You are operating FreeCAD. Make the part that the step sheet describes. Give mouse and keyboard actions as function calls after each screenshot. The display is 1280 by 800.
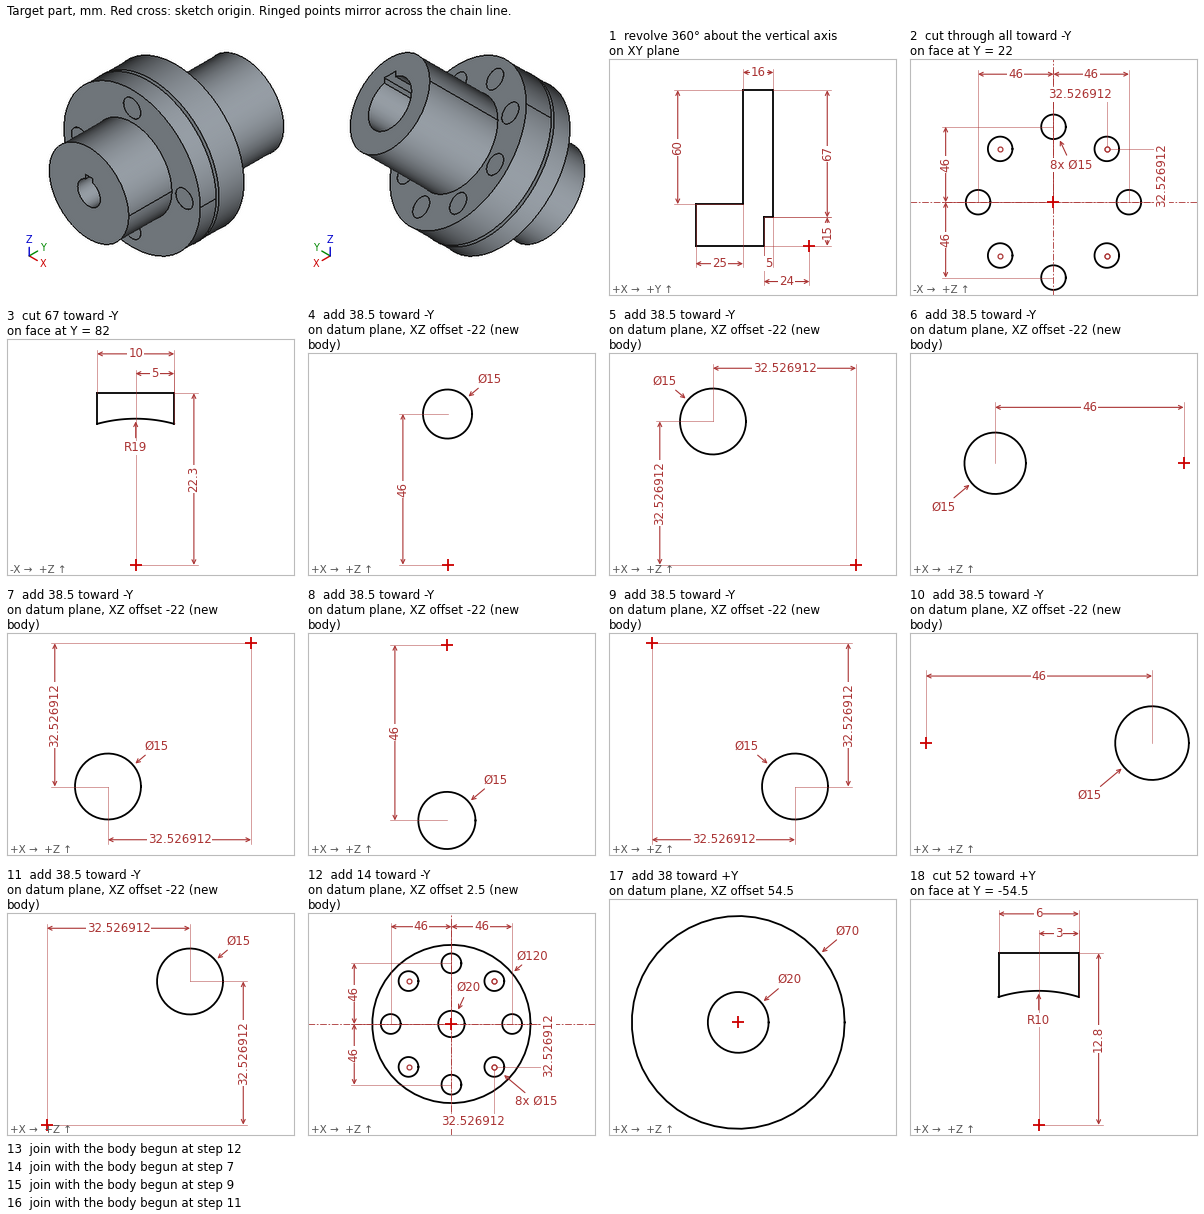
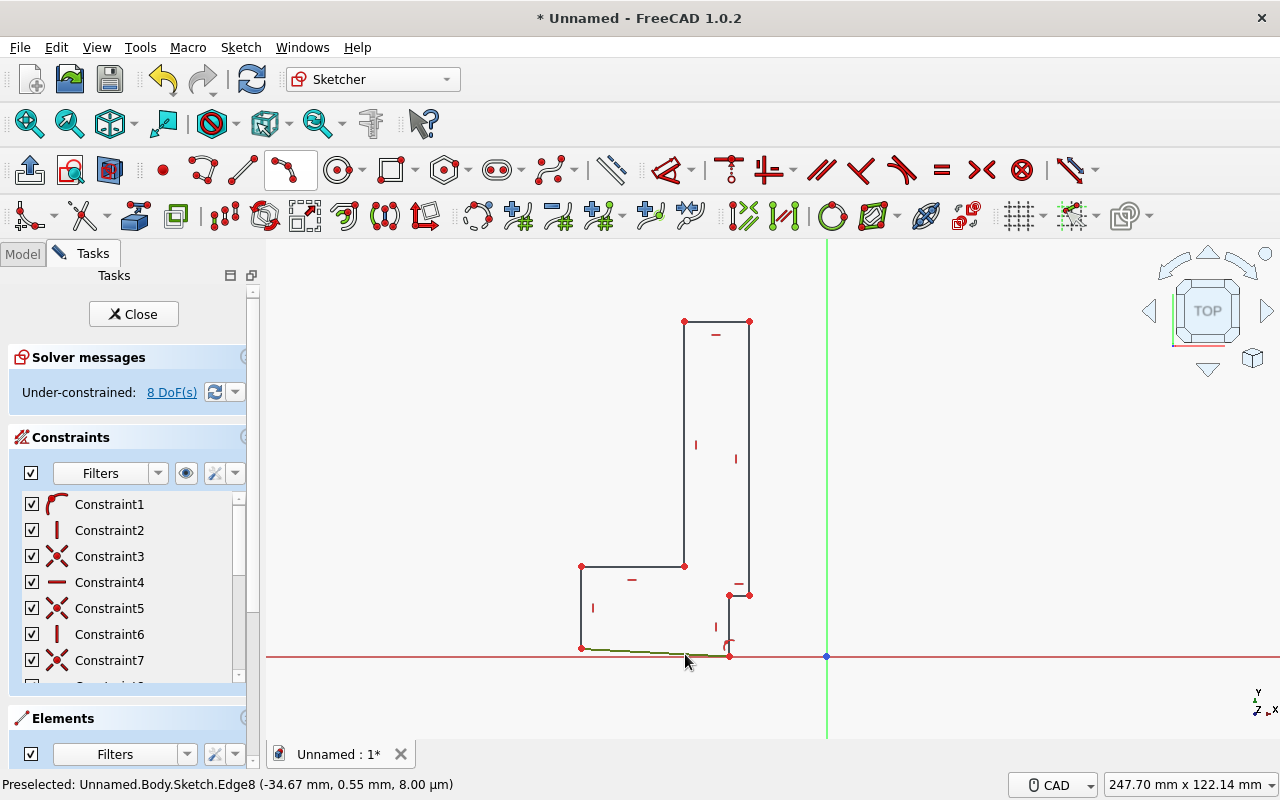
click(796, 170)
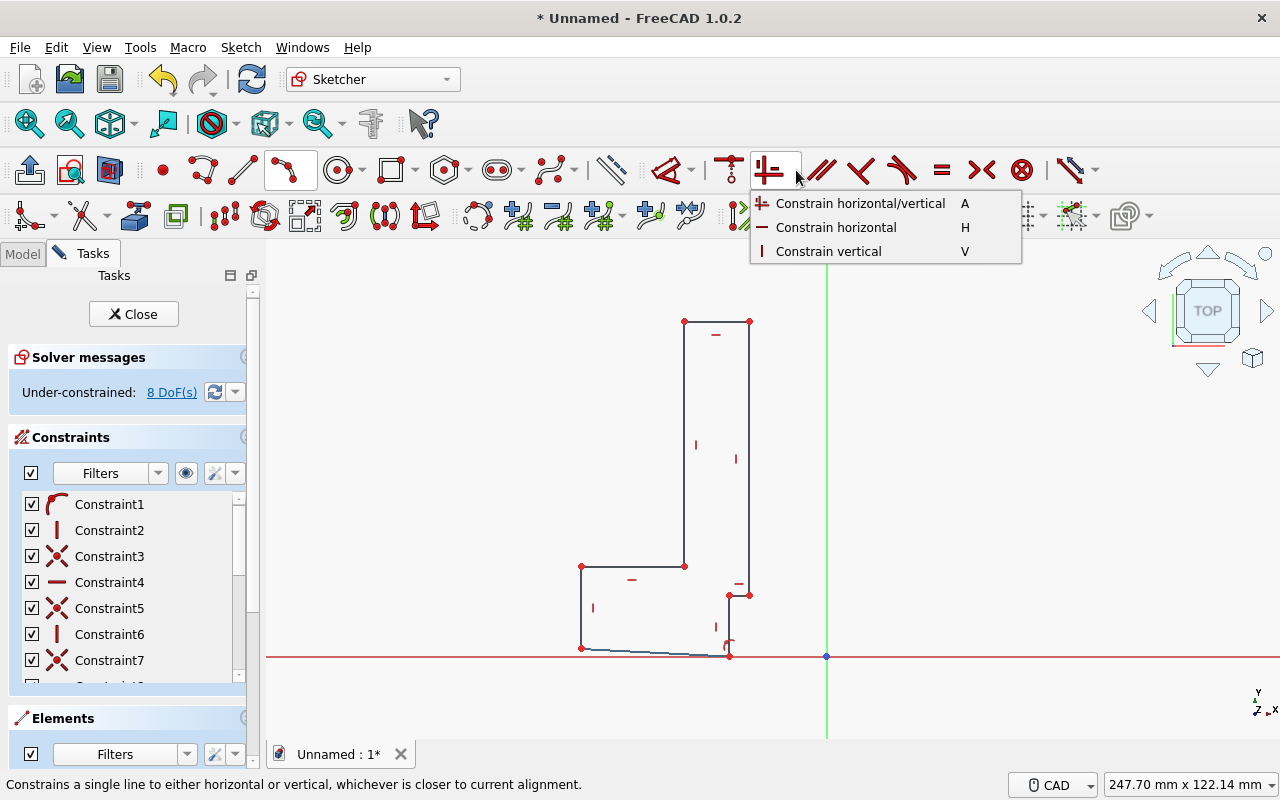
click(886, 227)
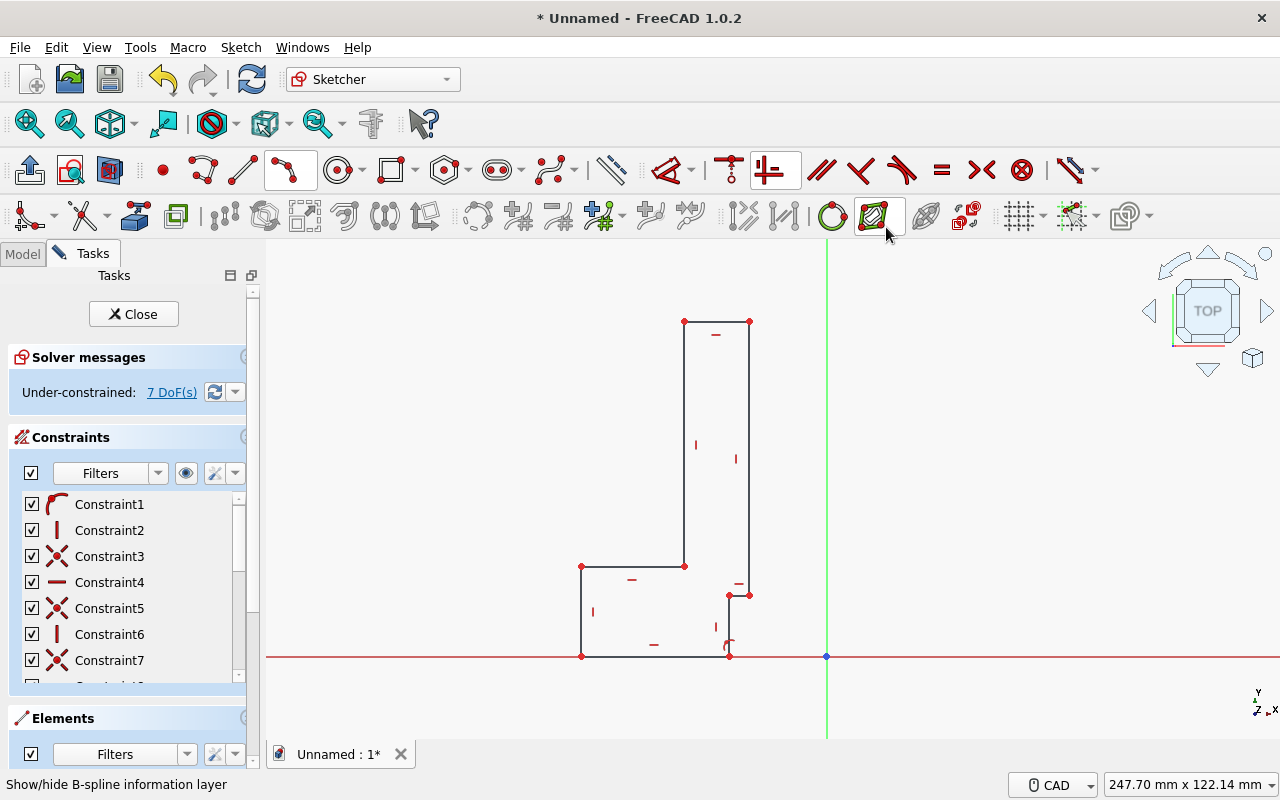
click(666, 170)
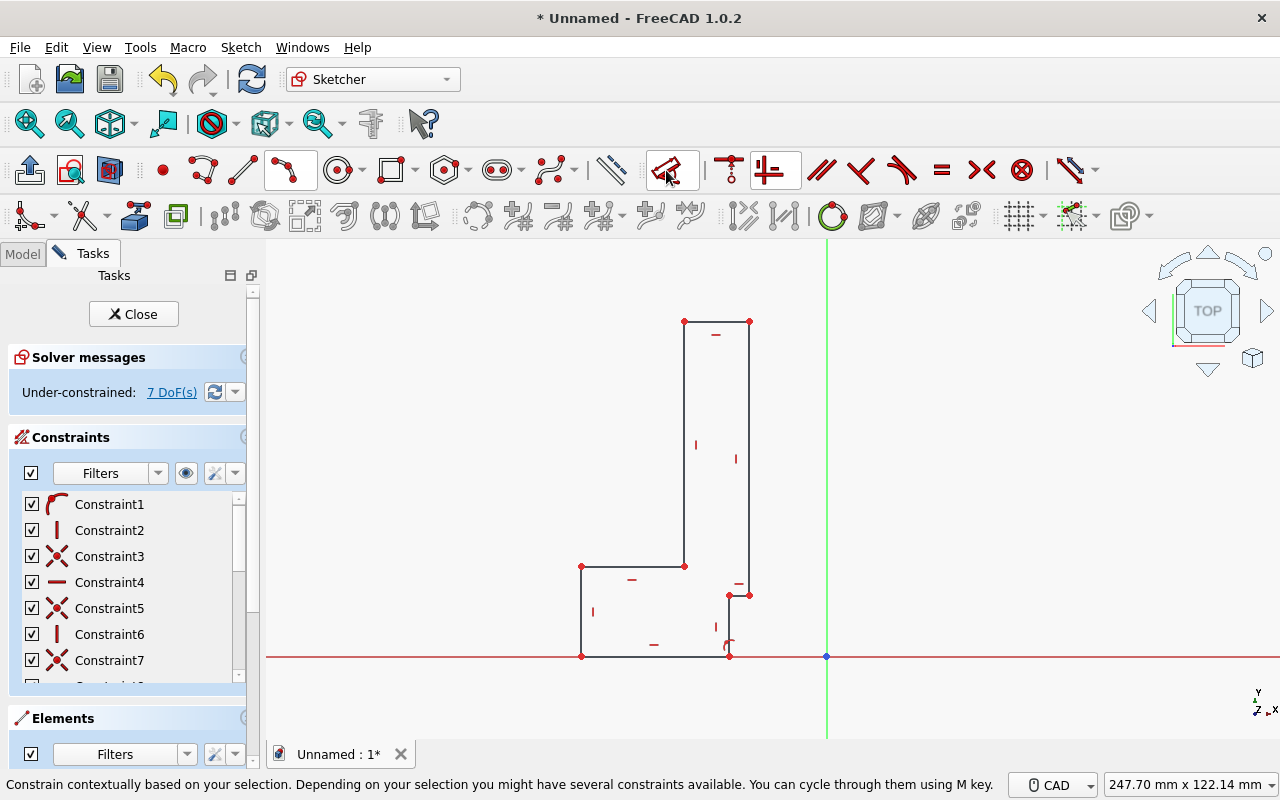
scroll(739, 596, up, 4)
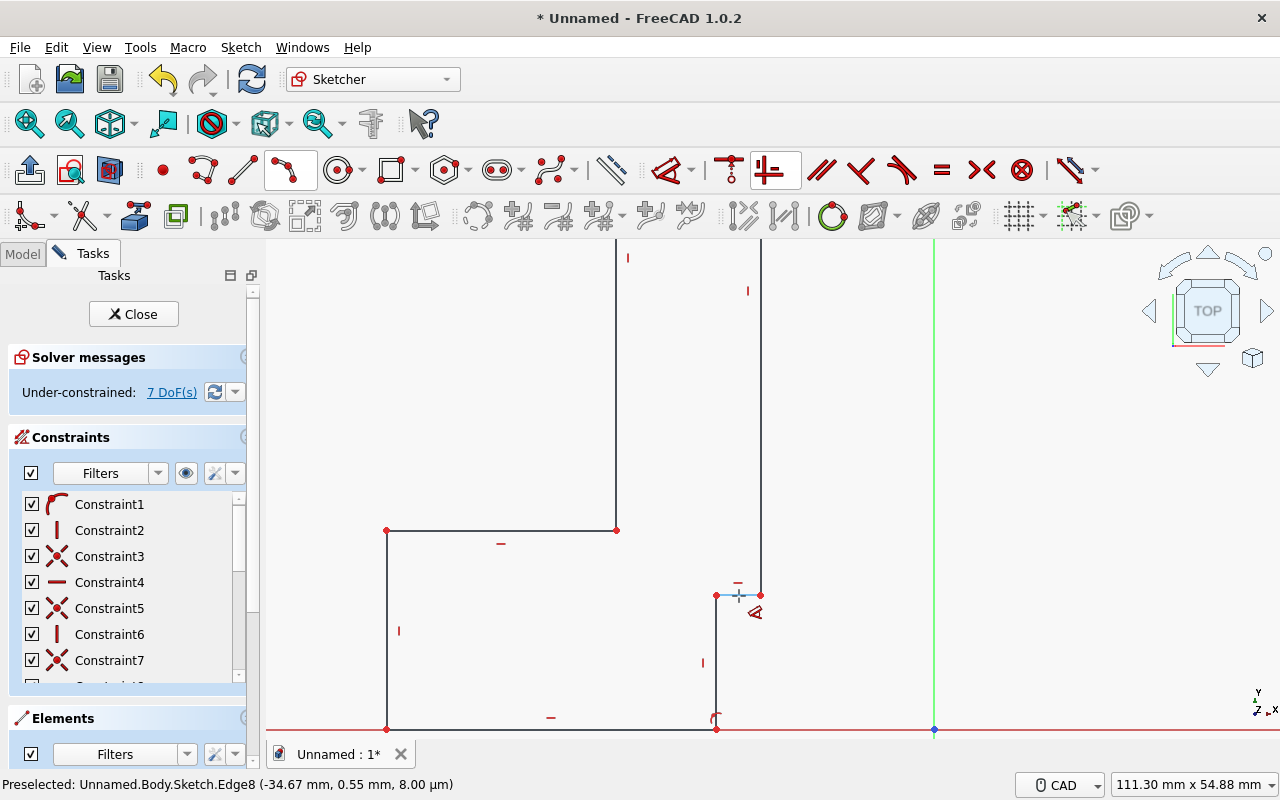
click(738, 595)
click(738, 629)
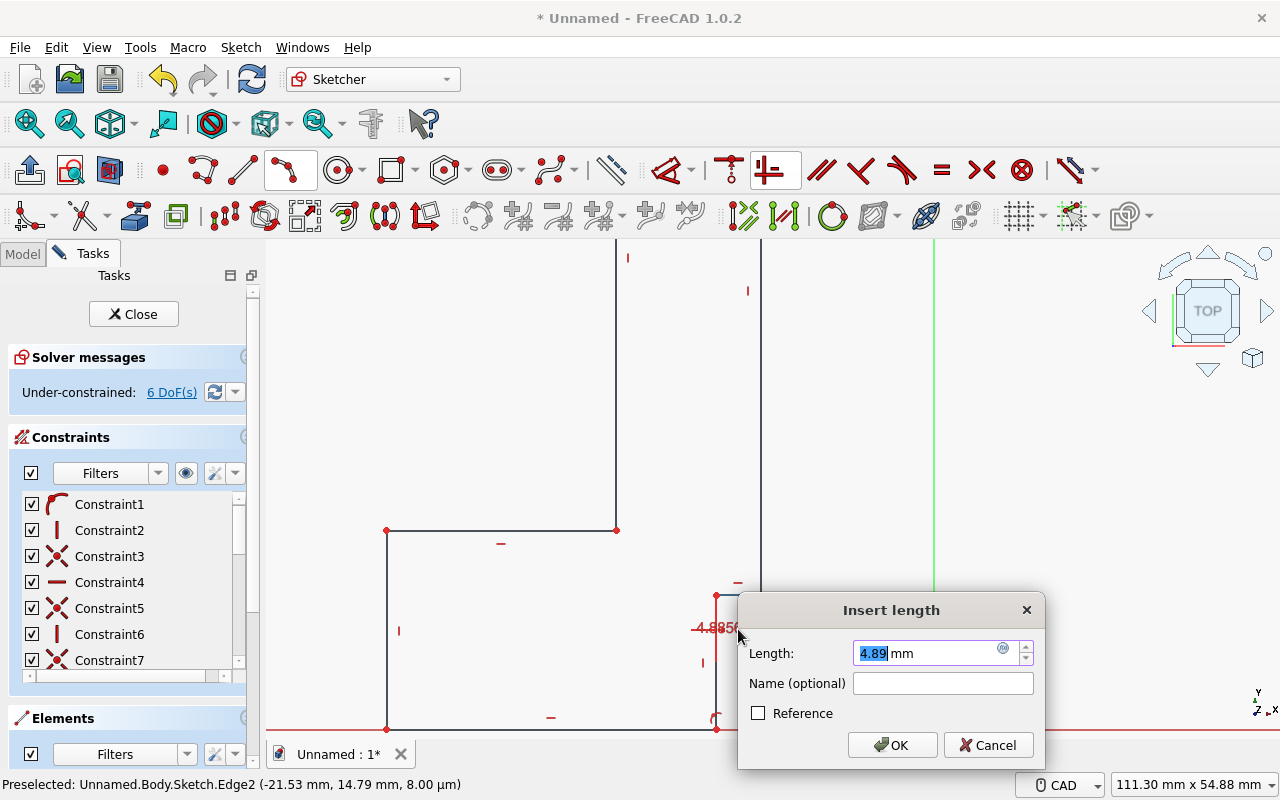
text(5)
key(Return)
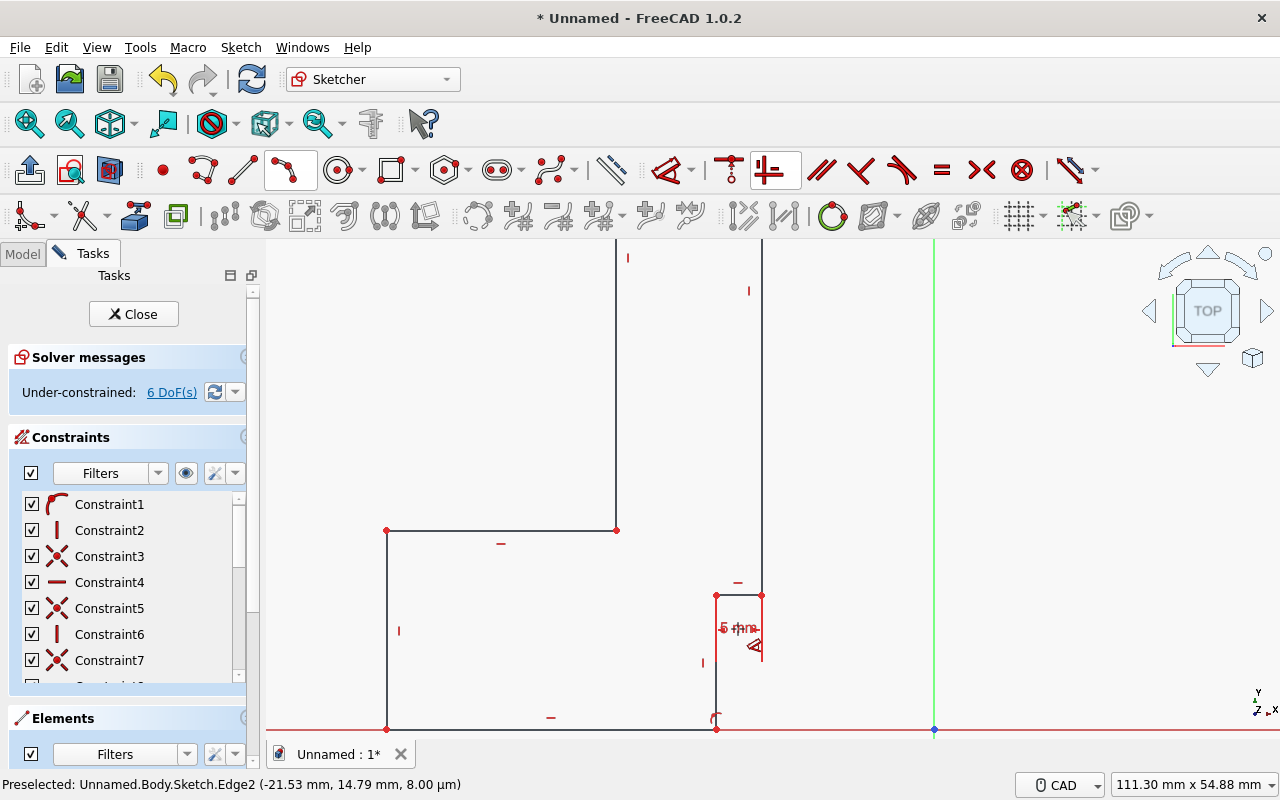
click(716, 689)
click(750, 653)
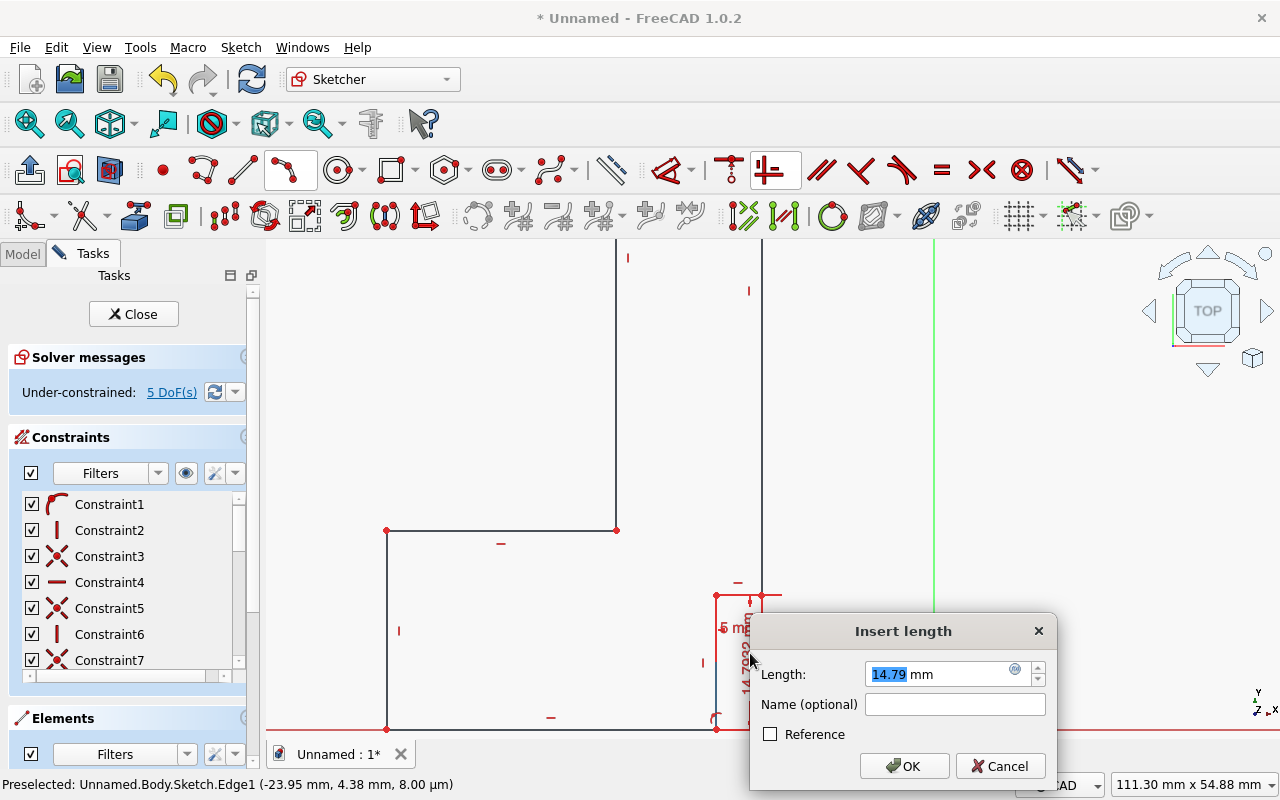
text(15)
key(Return)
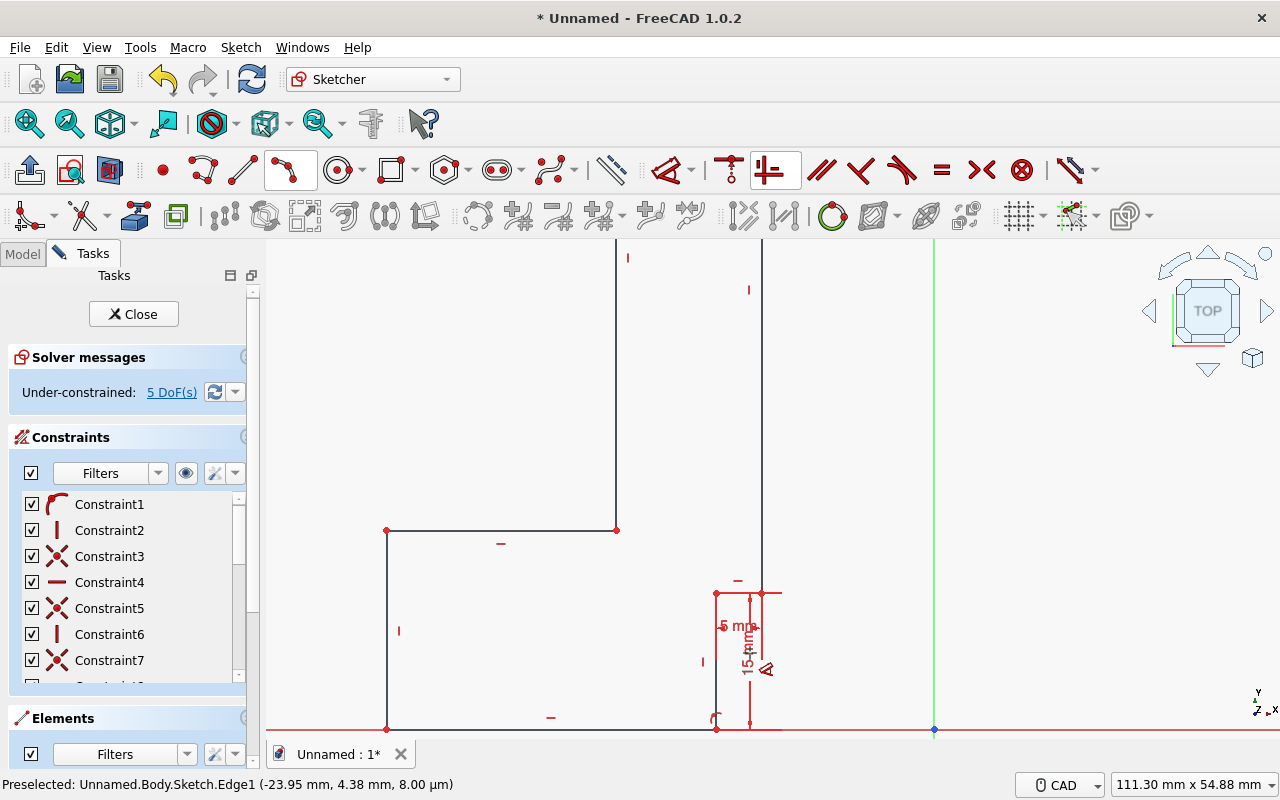
click(762, 411)
click(796, 430)